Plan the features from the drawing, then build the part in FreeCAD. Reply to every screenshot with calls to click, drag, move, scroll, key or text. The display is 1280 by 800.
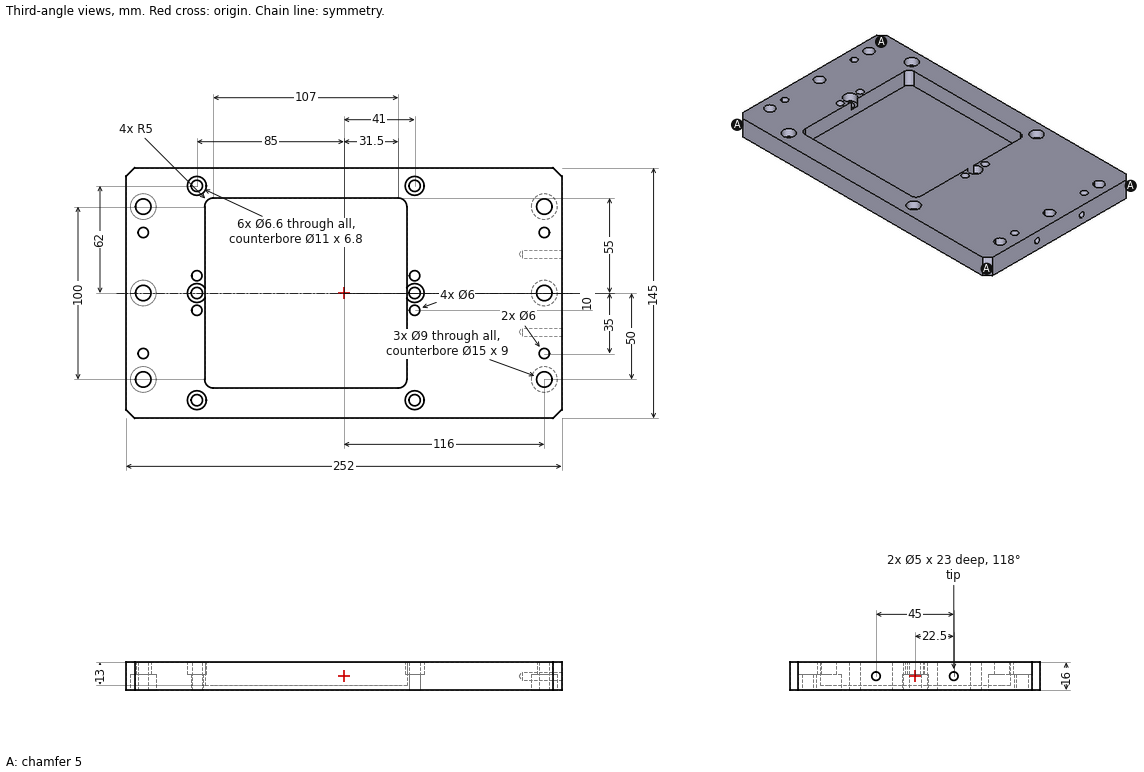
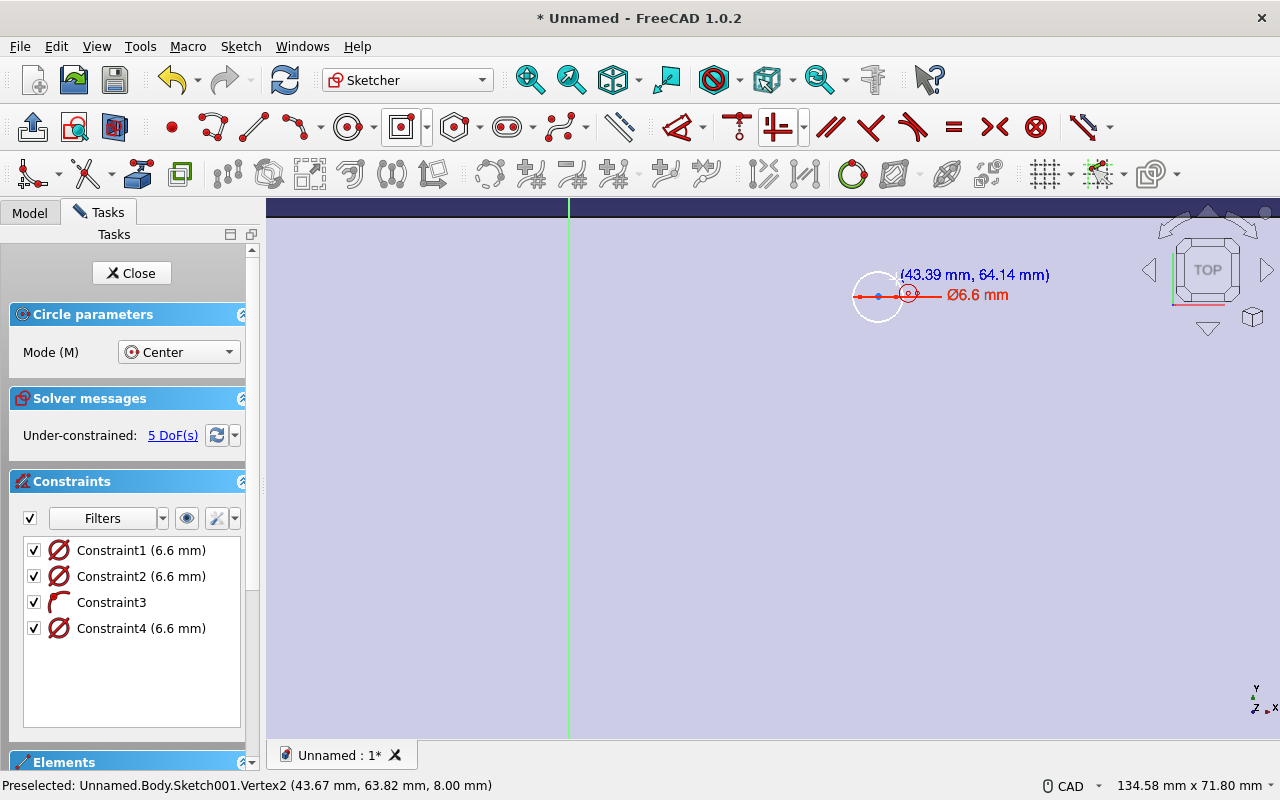
scroll(880, 297, down, 5)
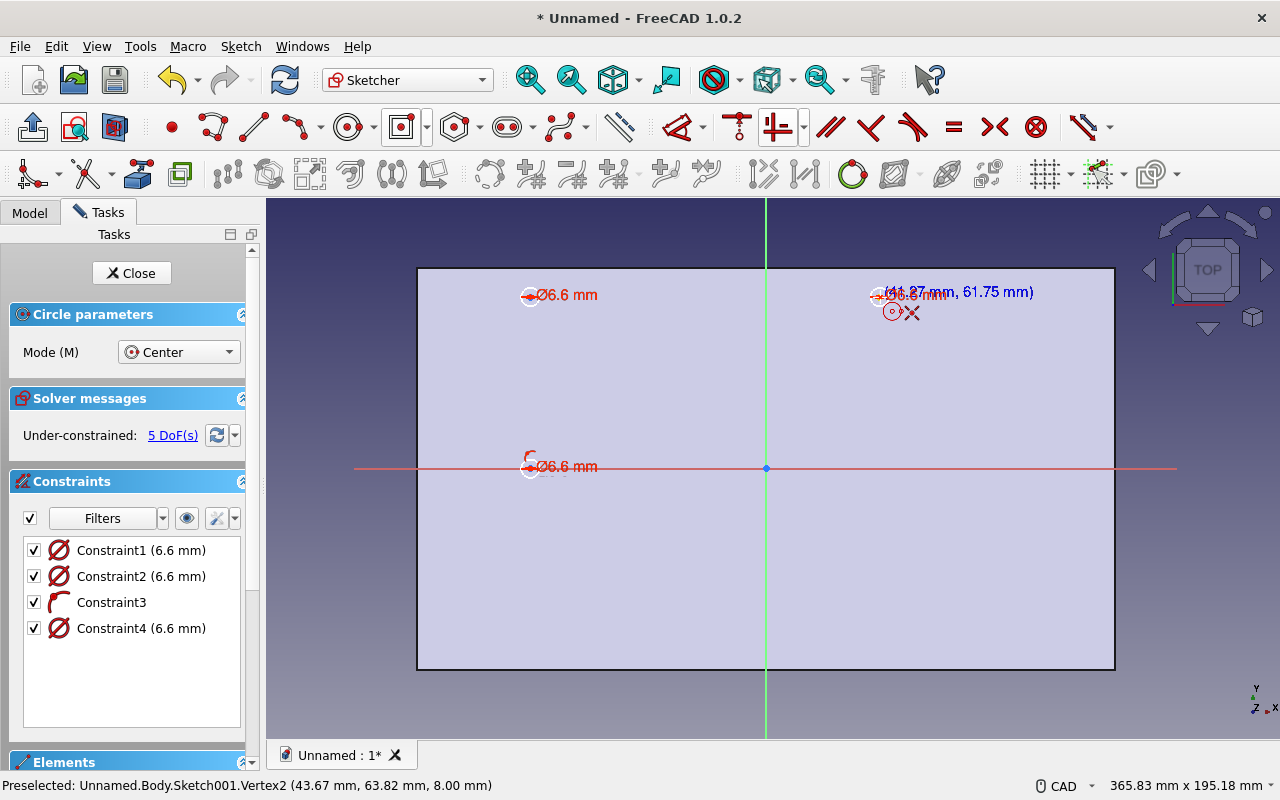
scroll(880, 469, up, 5)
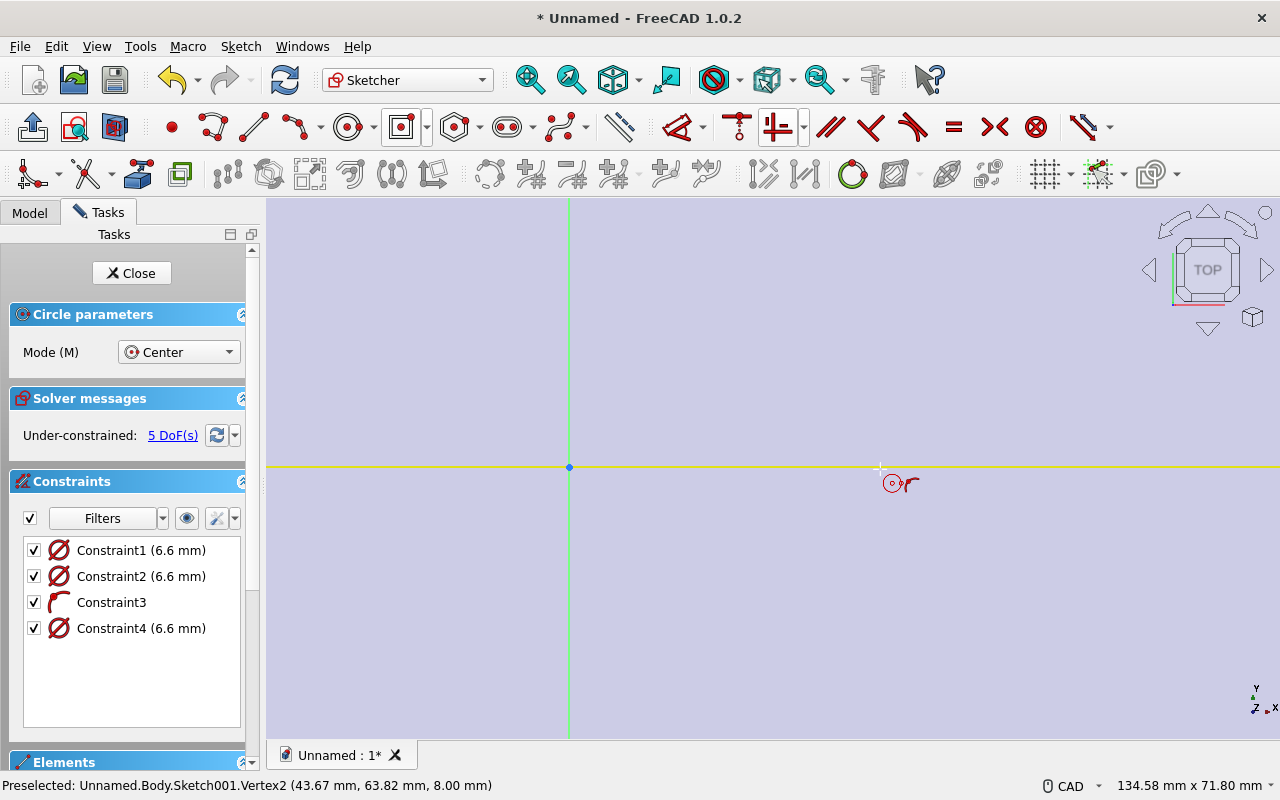
click(878, 467)
move(896, 450)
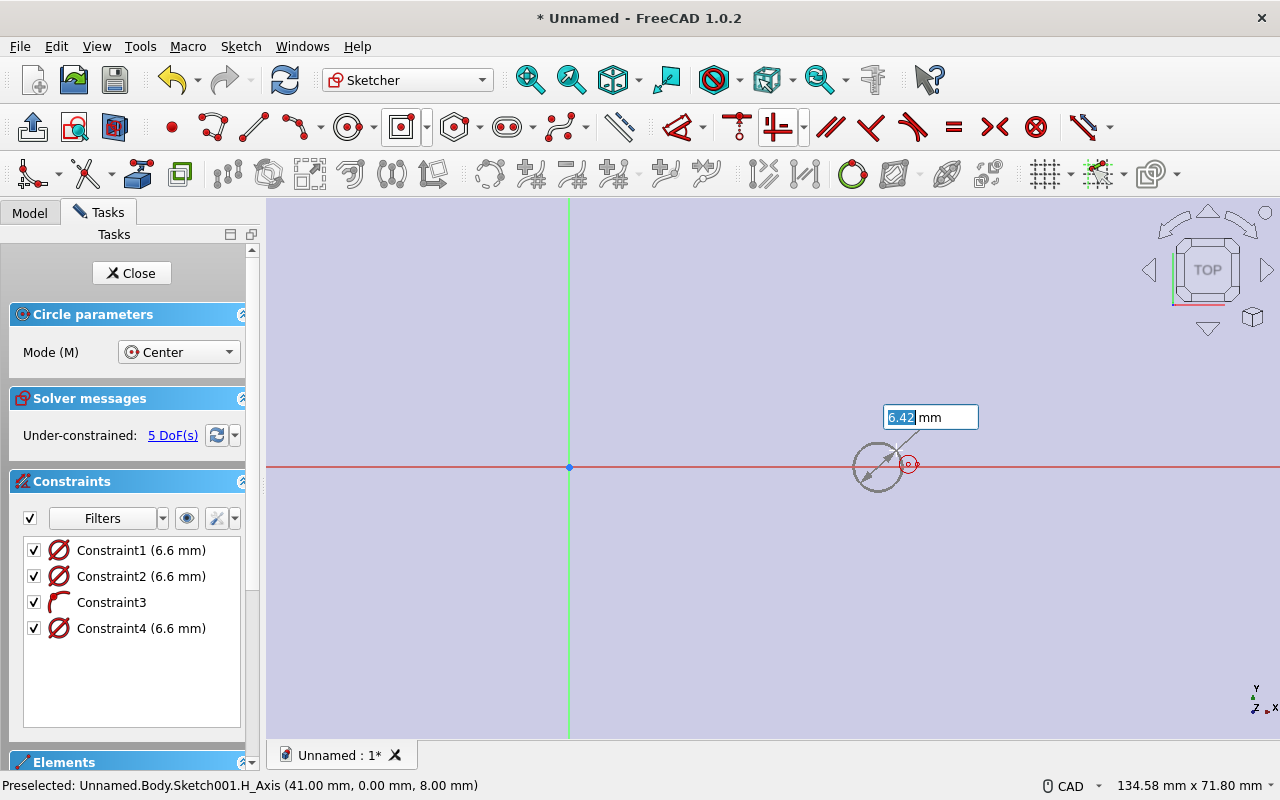
text(6.6)
key(Return)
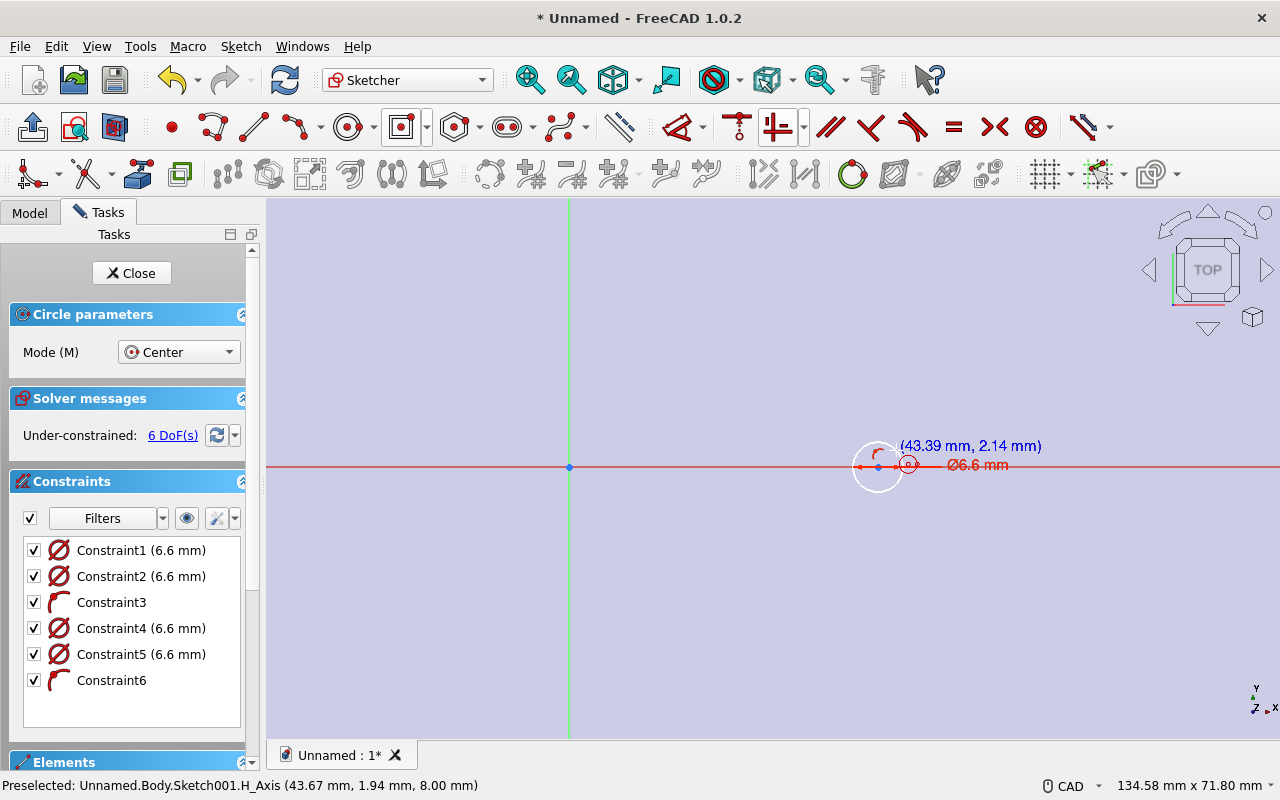
scroll(880, 469, down, 5)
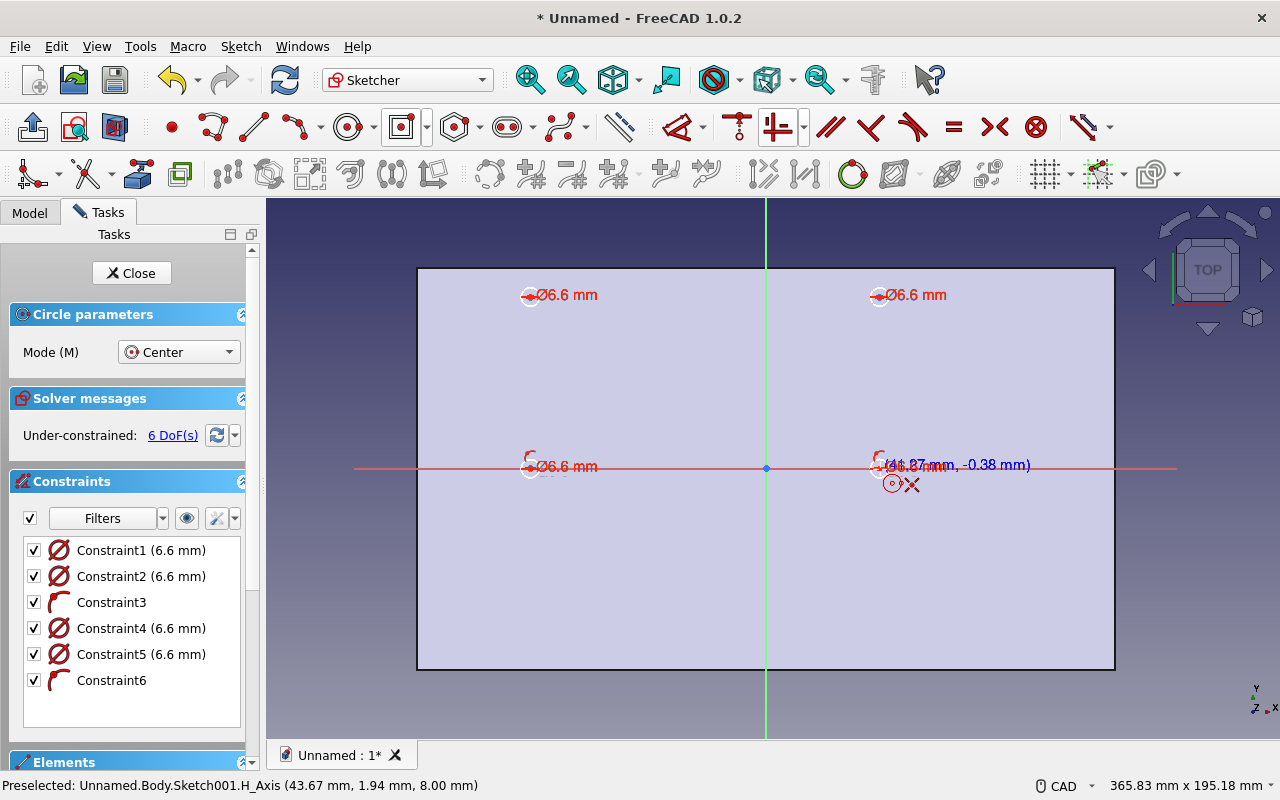
scroll(880, 640, up, 5)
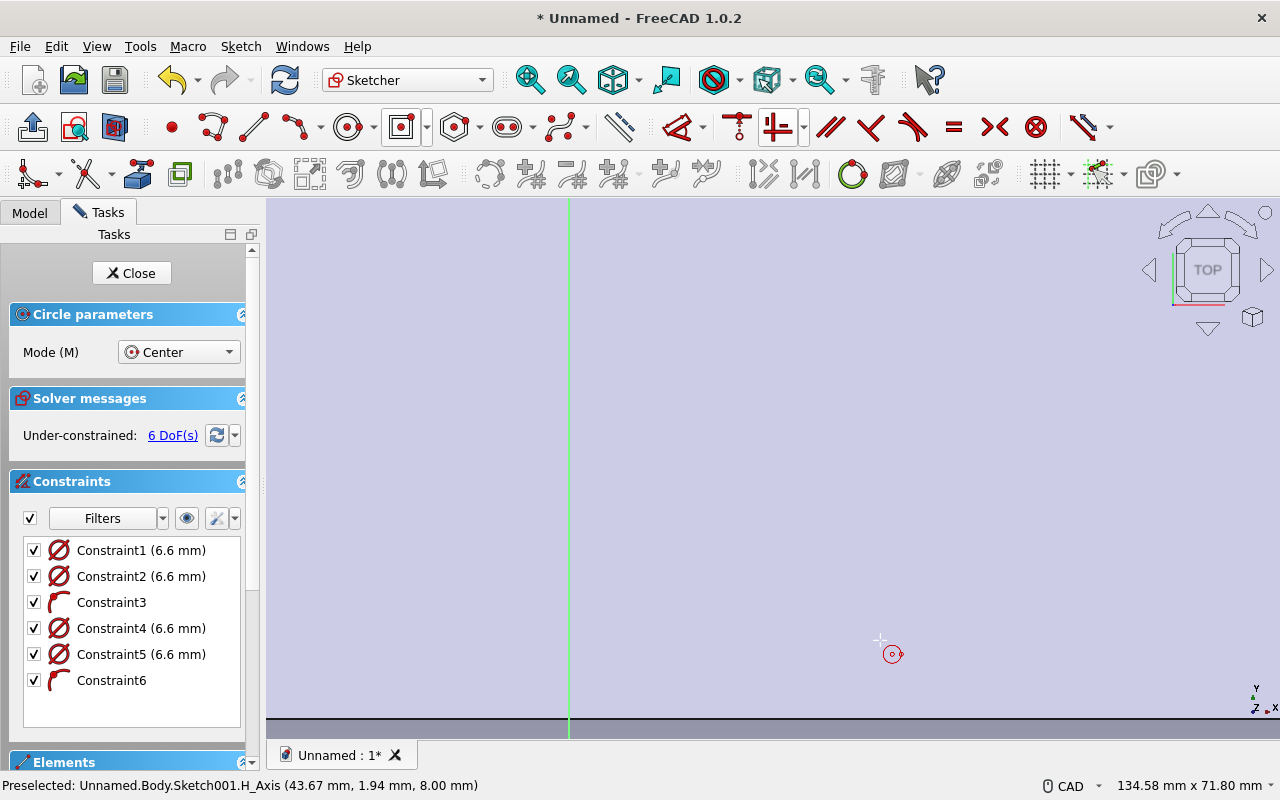
click(878, 640)
move(896, 622)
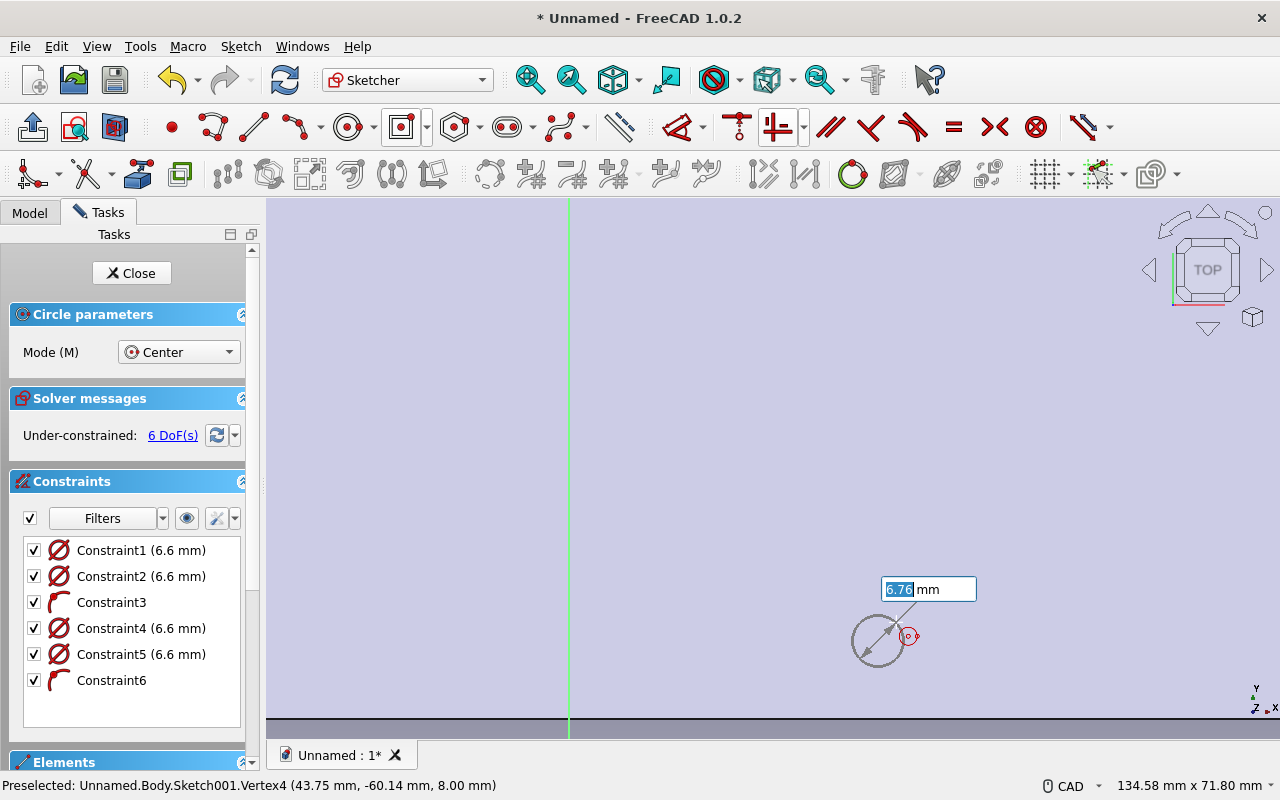
text(6.6)
key(Return)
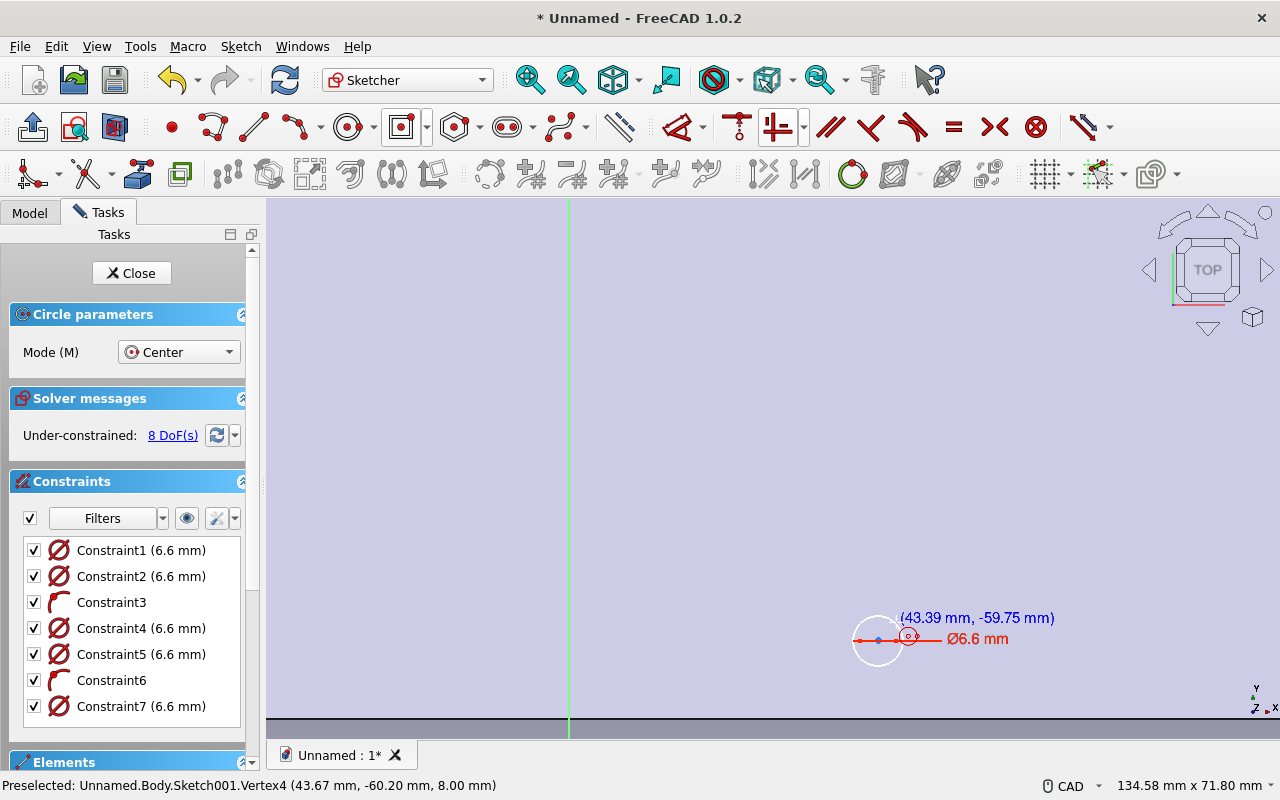
scroll(880, 641, down, 5)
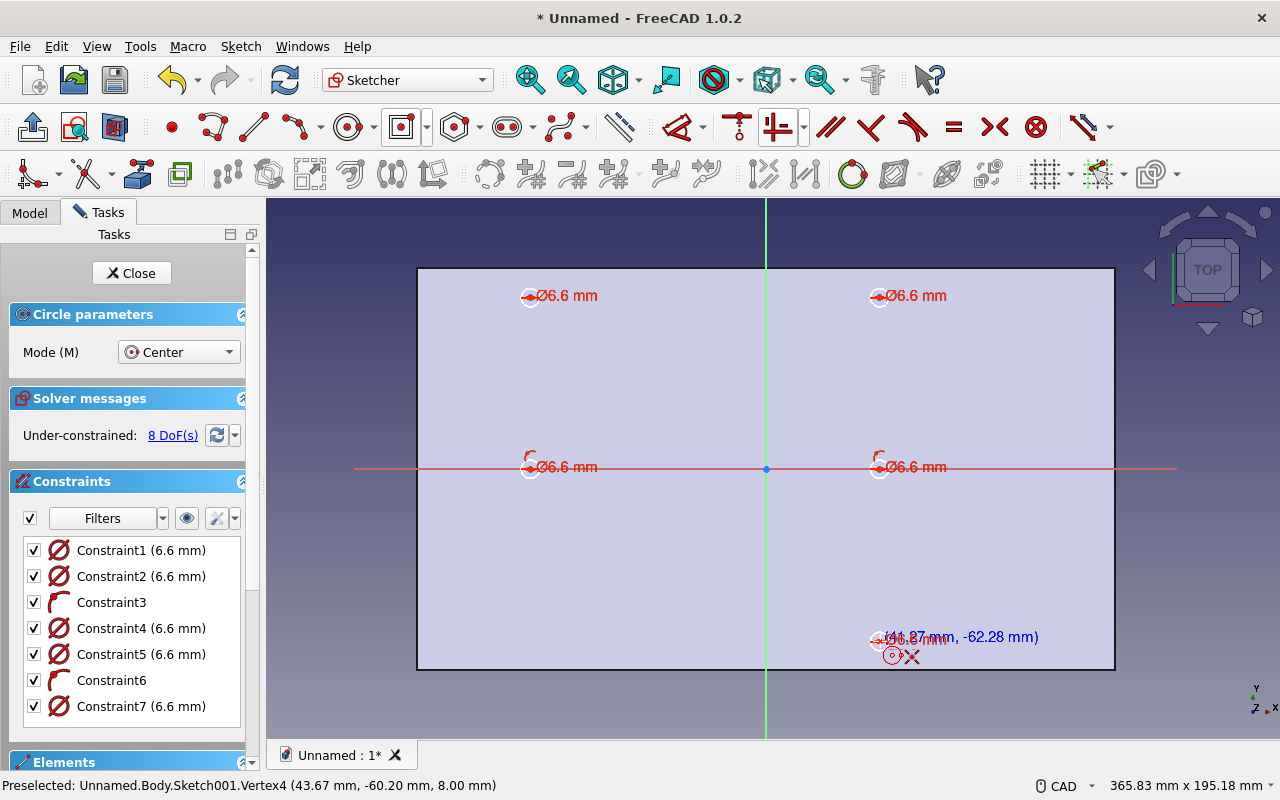
scroll(530, 641, up, 5)